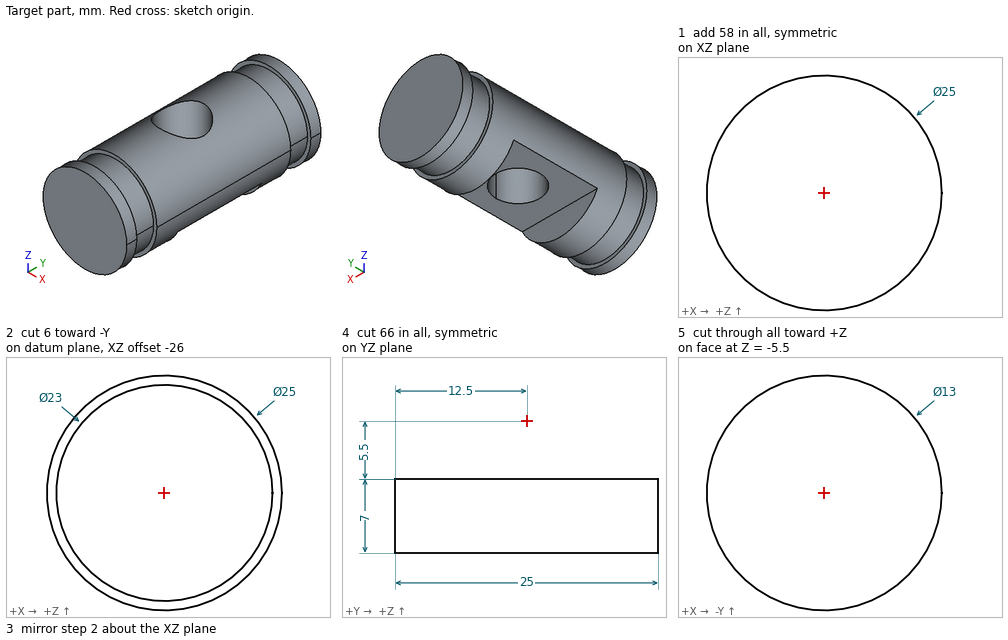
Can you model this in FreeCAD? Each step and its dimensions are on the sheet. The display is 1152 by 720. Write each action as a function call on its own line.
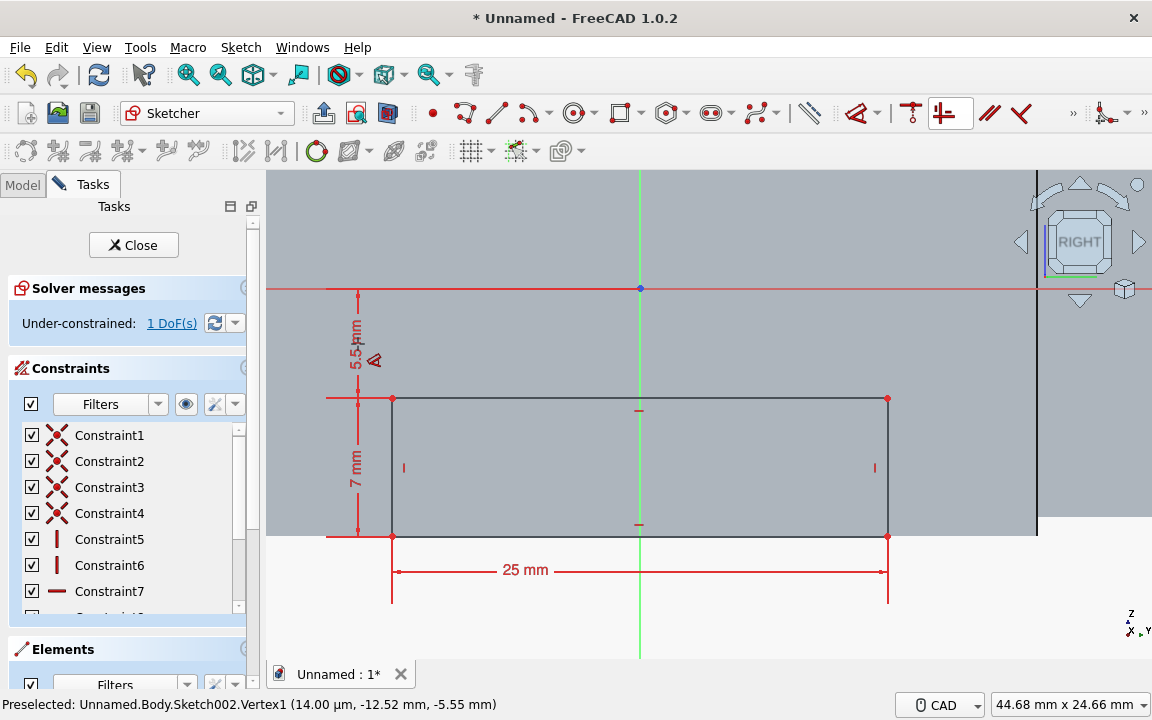
click(392, 398)
click(516, 255)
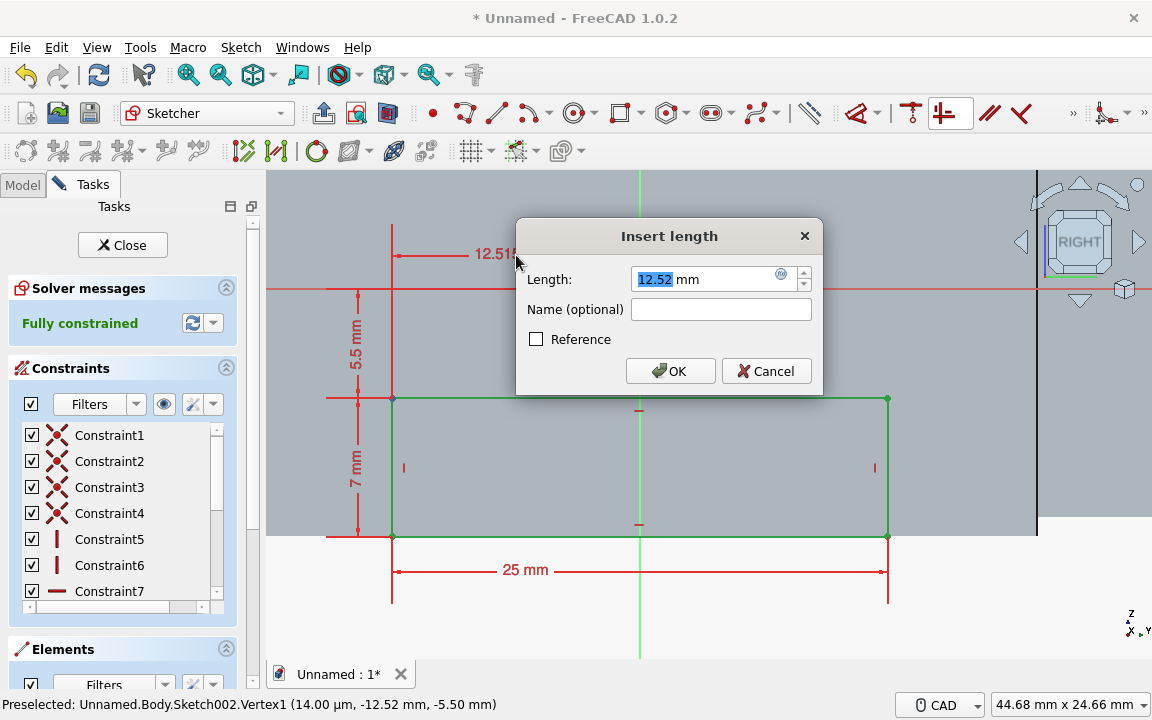
text(12.5)
key(Return)
key(Escape)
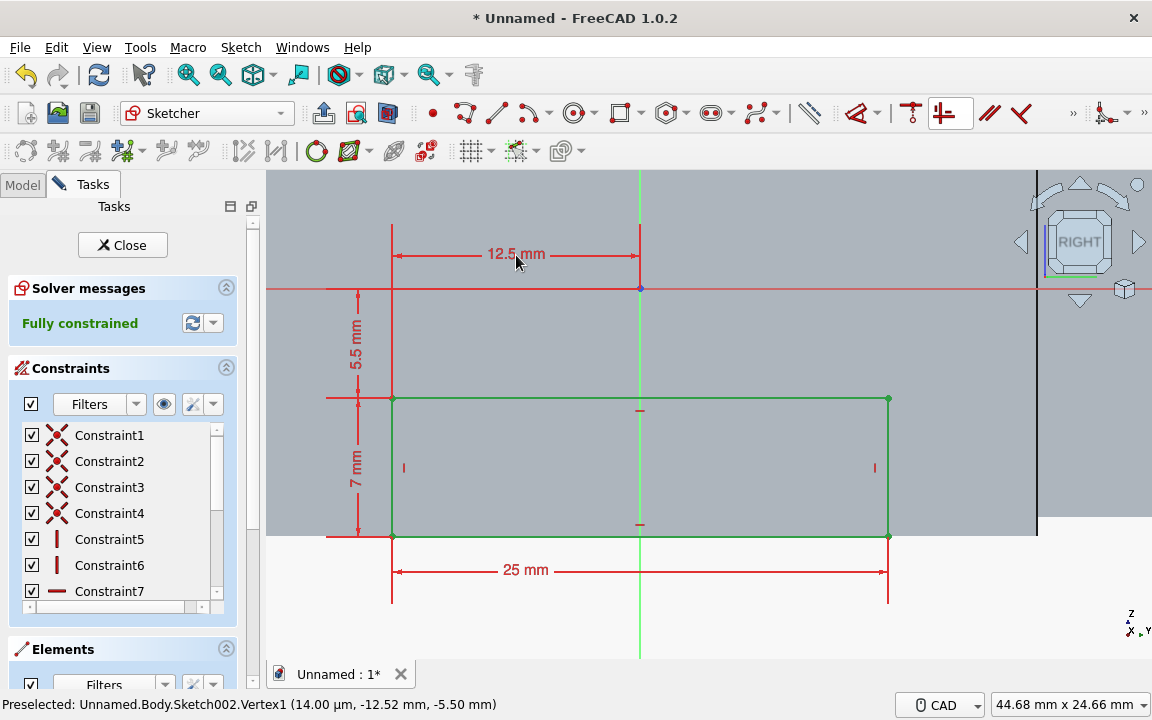
click(123, 245)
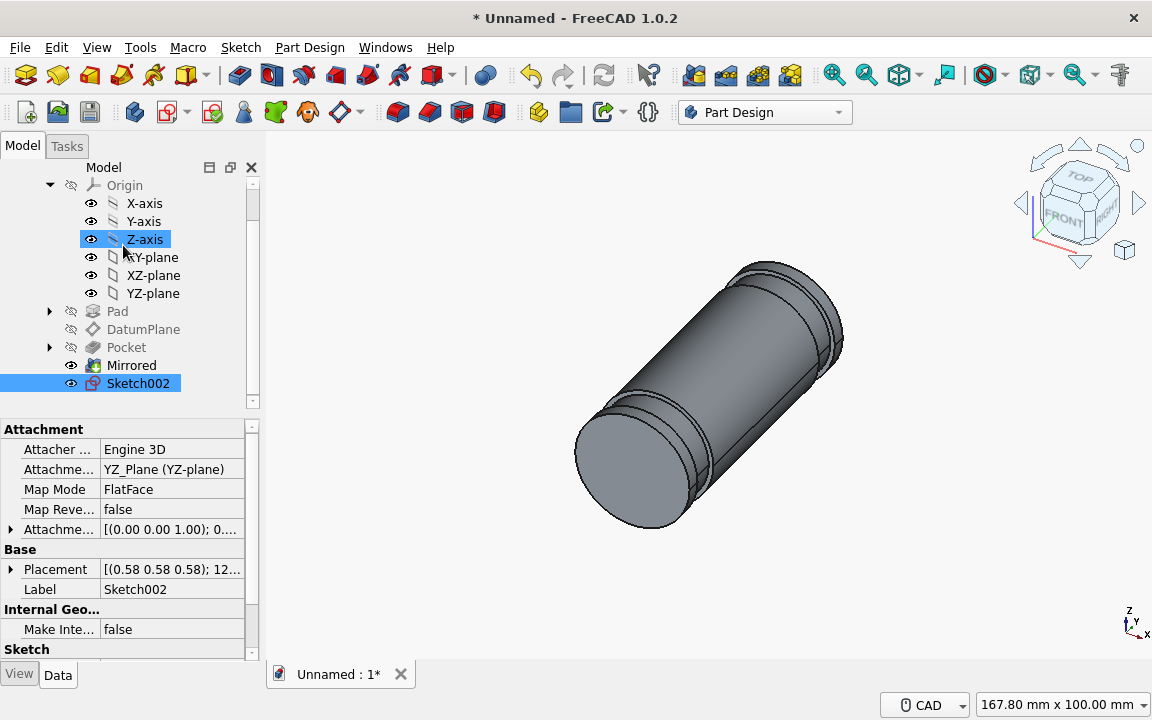
click(240, 76)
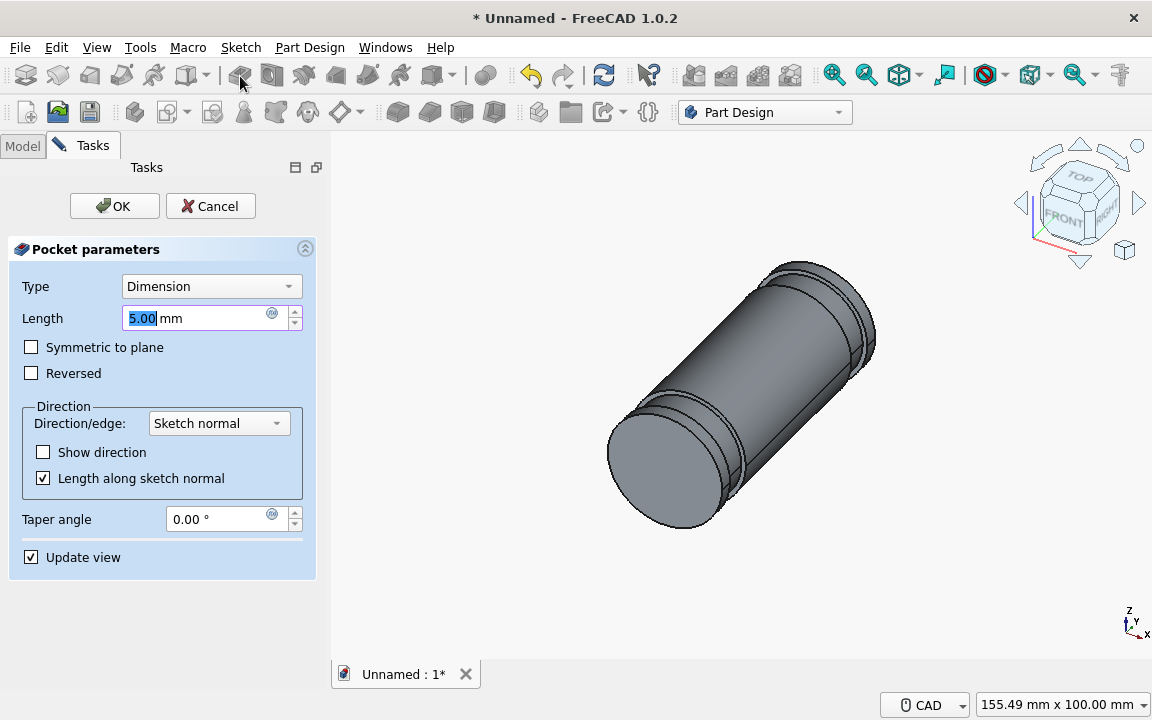
text(66)
key(Tab)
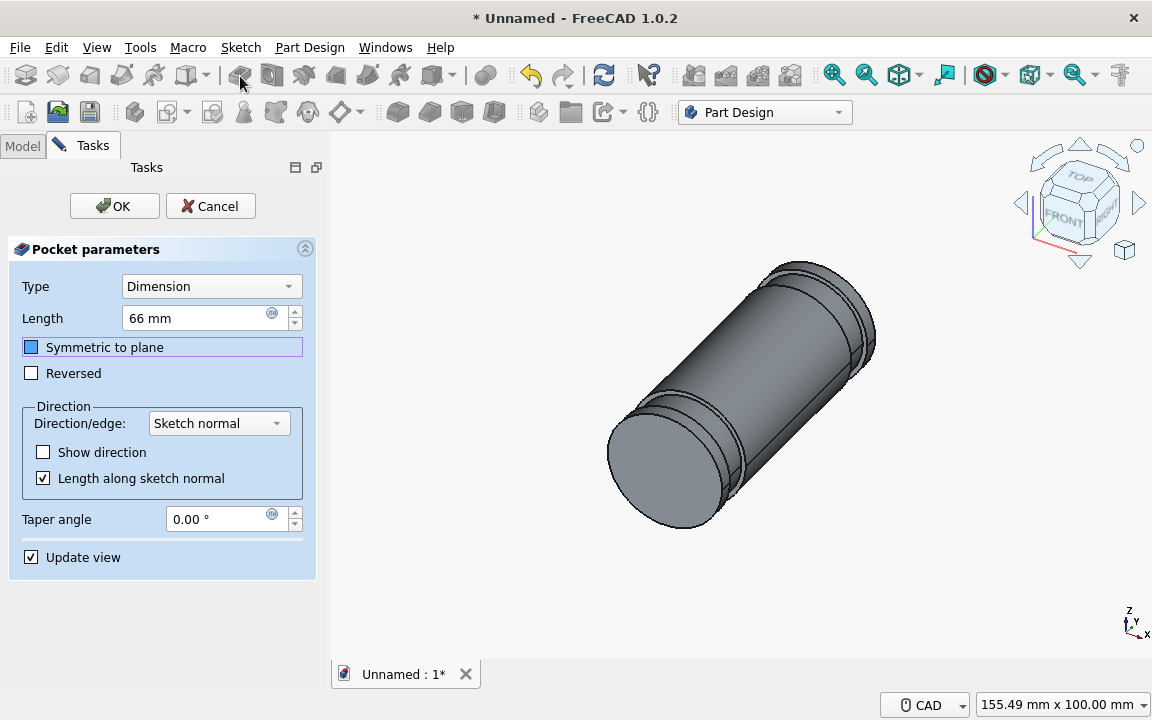
click(30, 347)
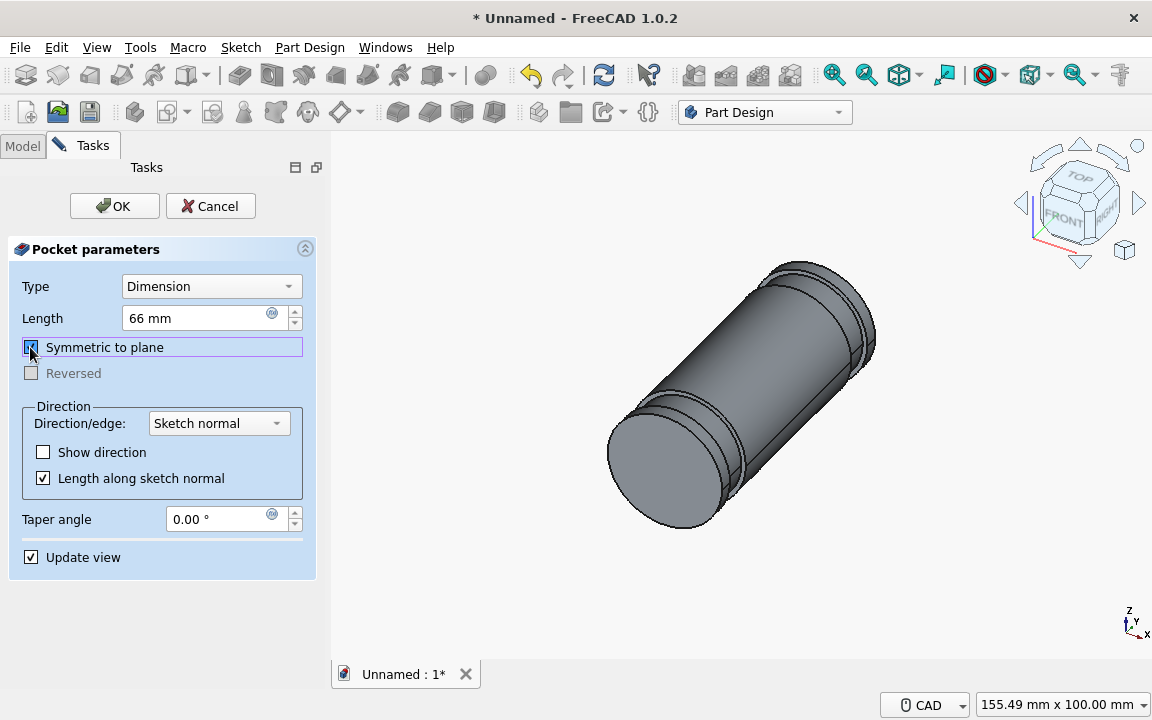
click(115, 206)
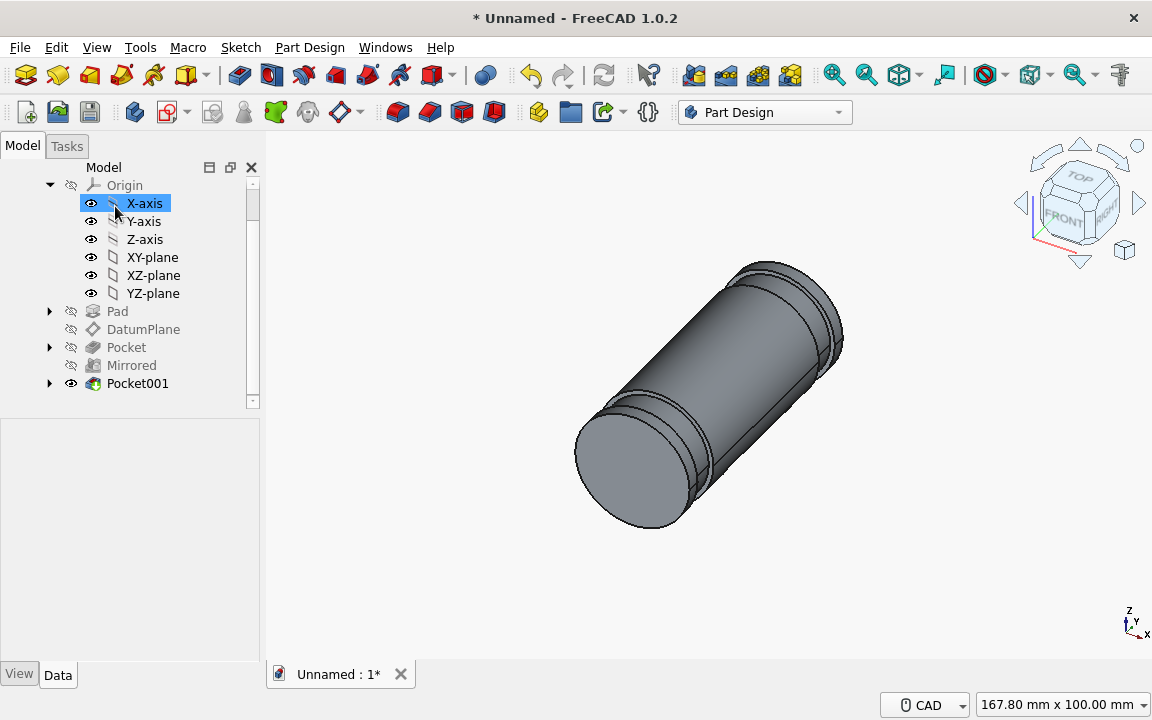
key(5)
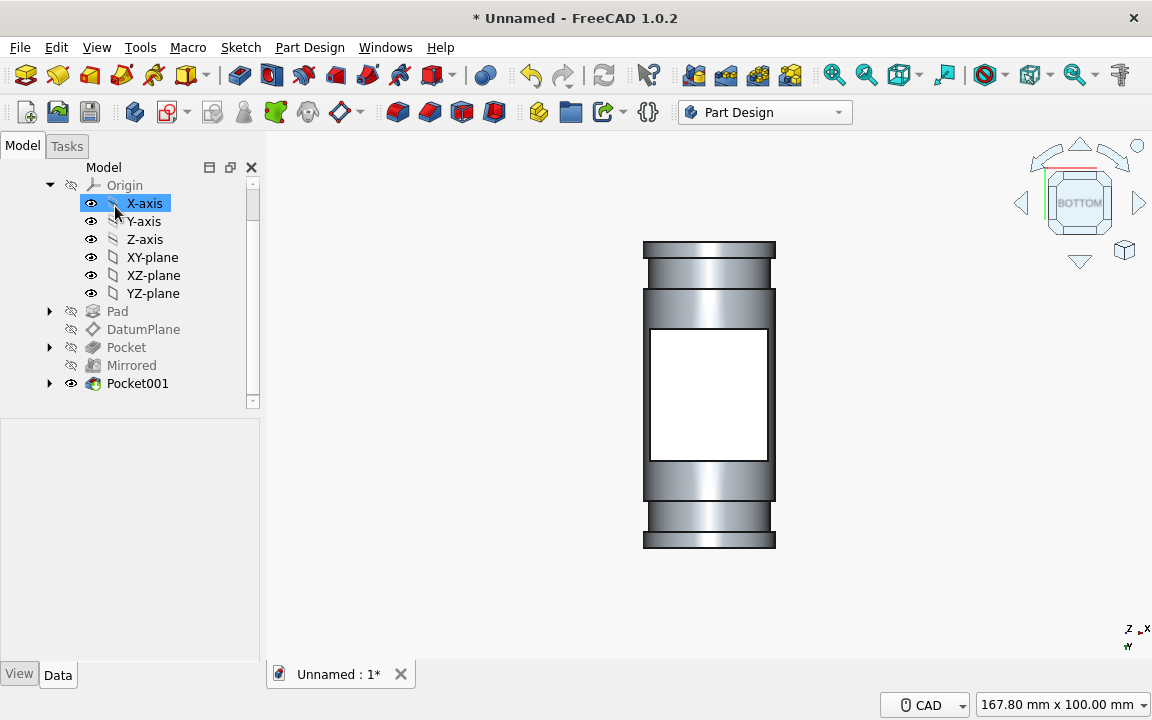
click(709, 394)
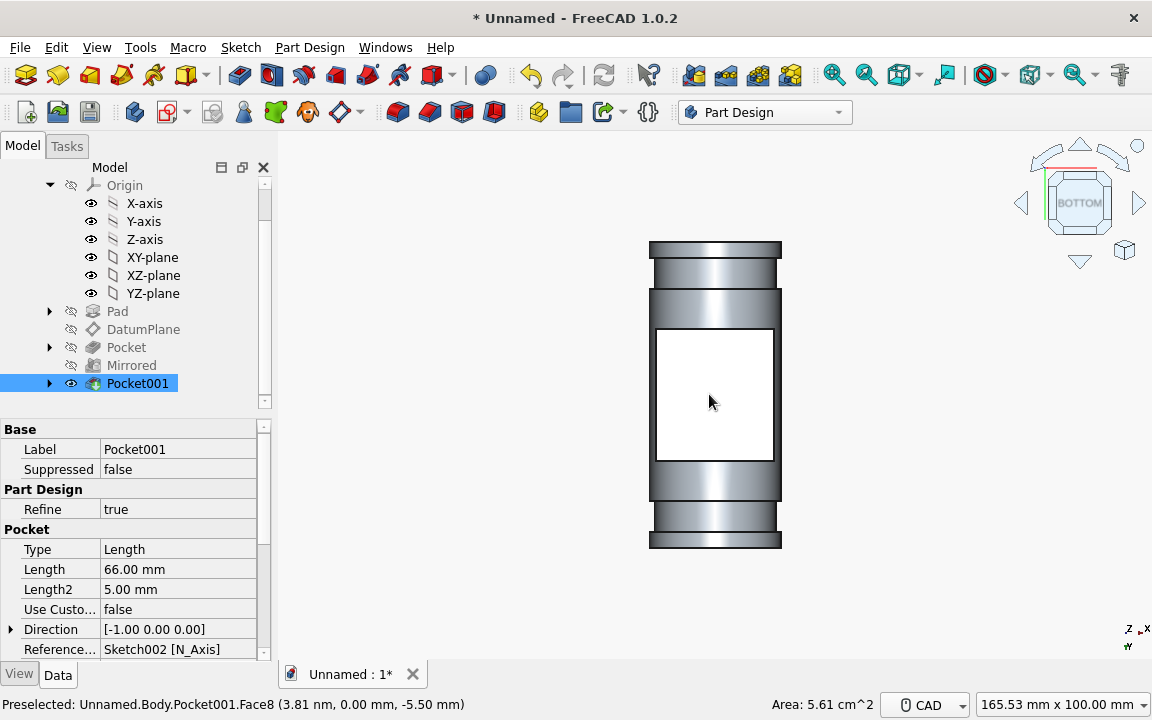
click(168, 112)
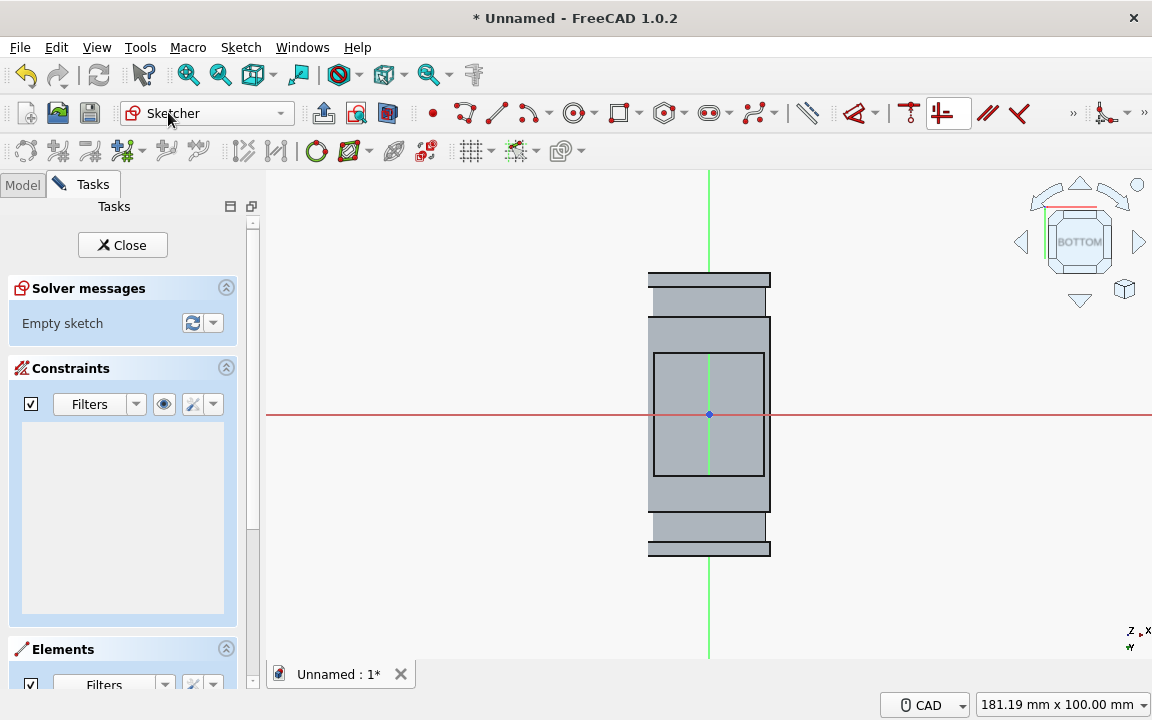
click(388, 114)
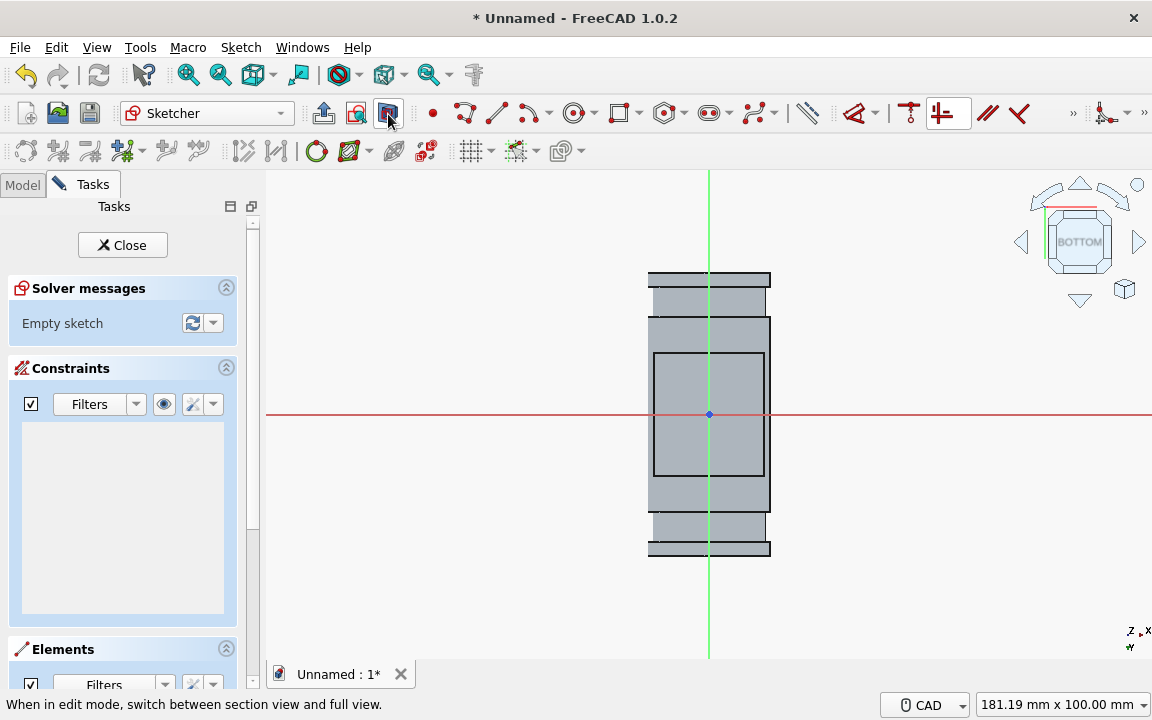
scroll(726, 414, up, 8)